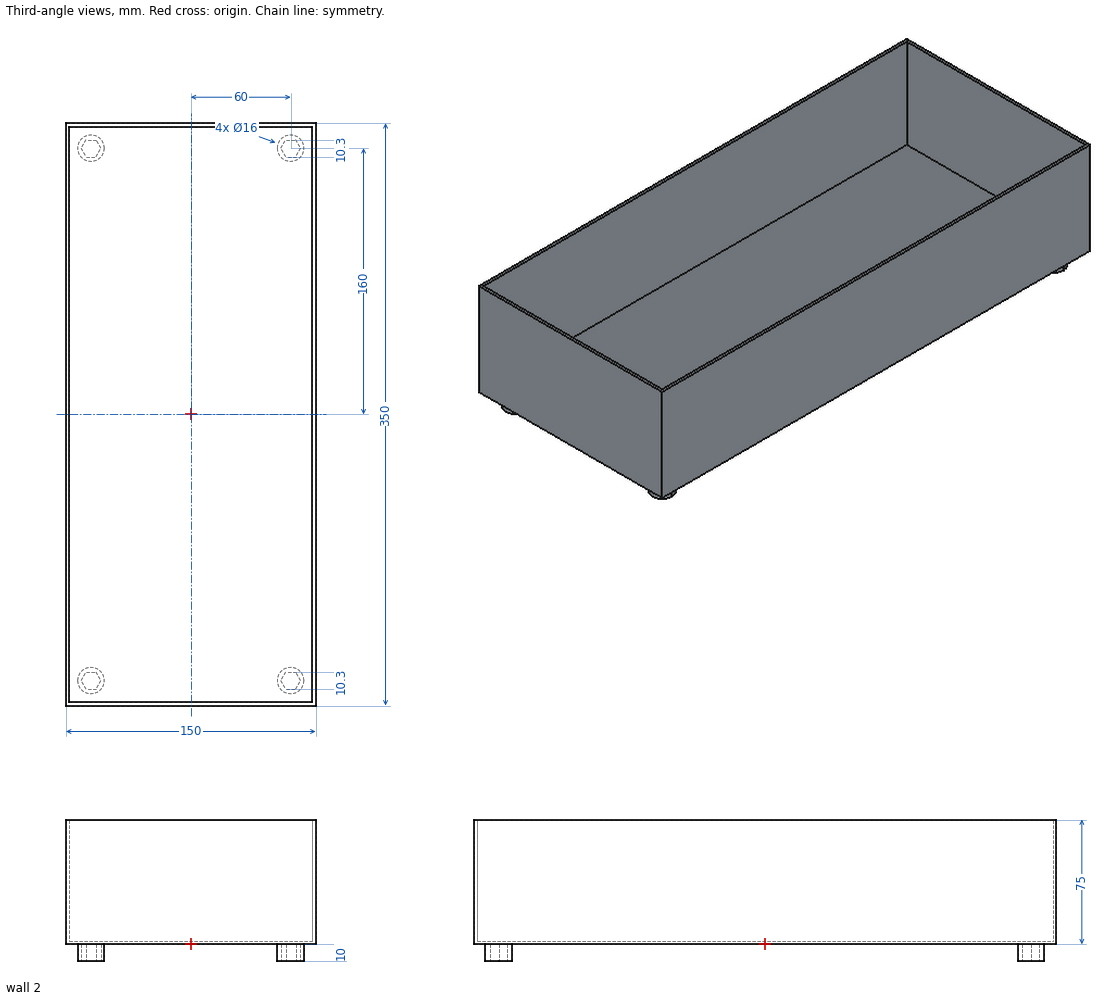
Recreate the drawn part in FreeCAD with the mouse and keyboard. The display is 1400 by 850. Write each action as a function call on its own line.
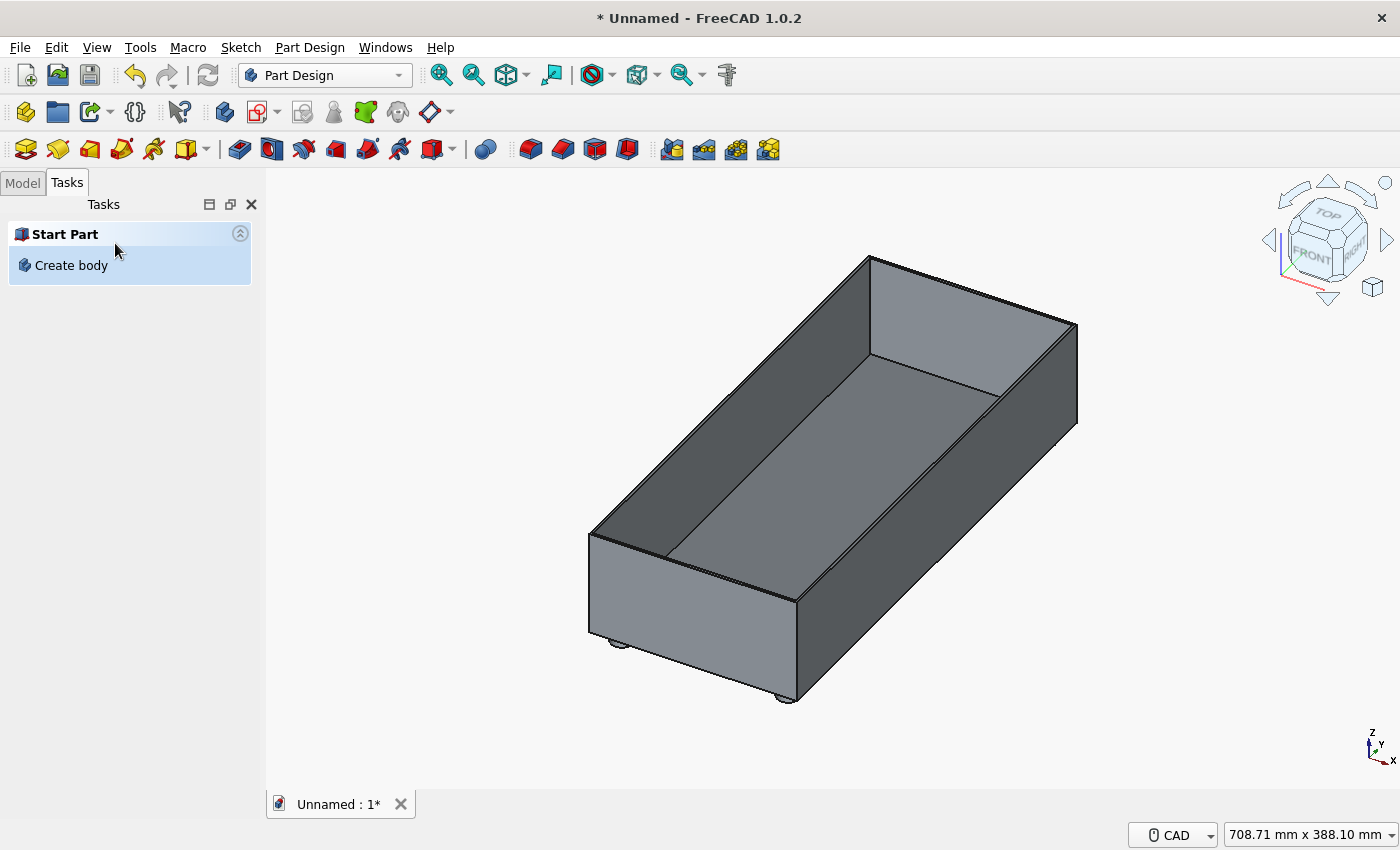
key(0)